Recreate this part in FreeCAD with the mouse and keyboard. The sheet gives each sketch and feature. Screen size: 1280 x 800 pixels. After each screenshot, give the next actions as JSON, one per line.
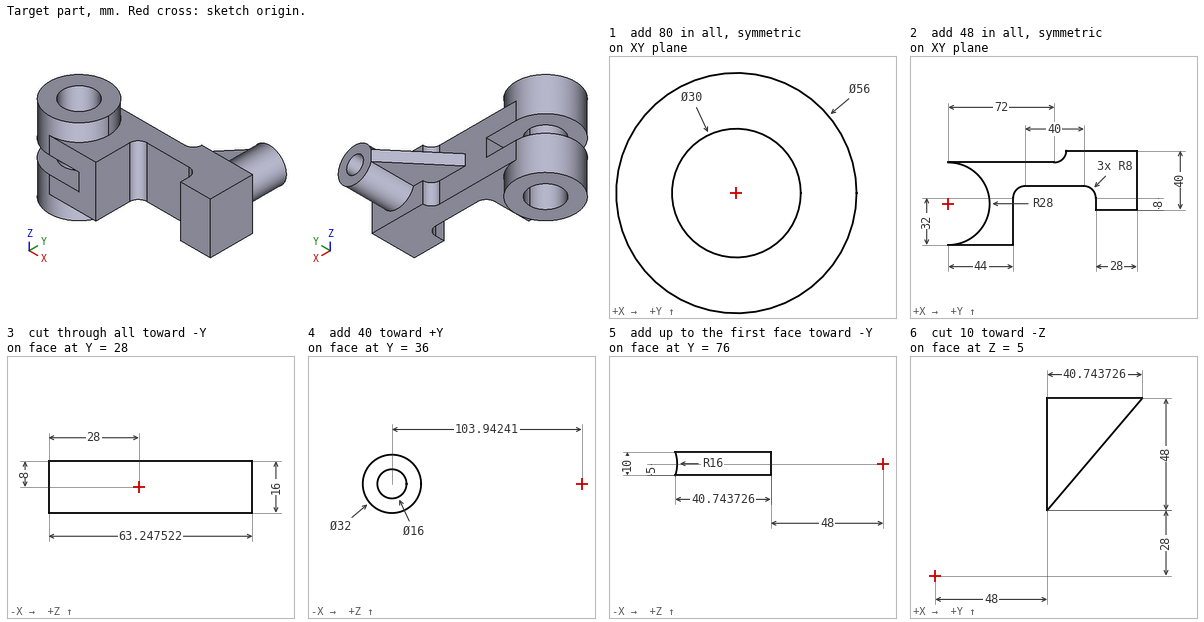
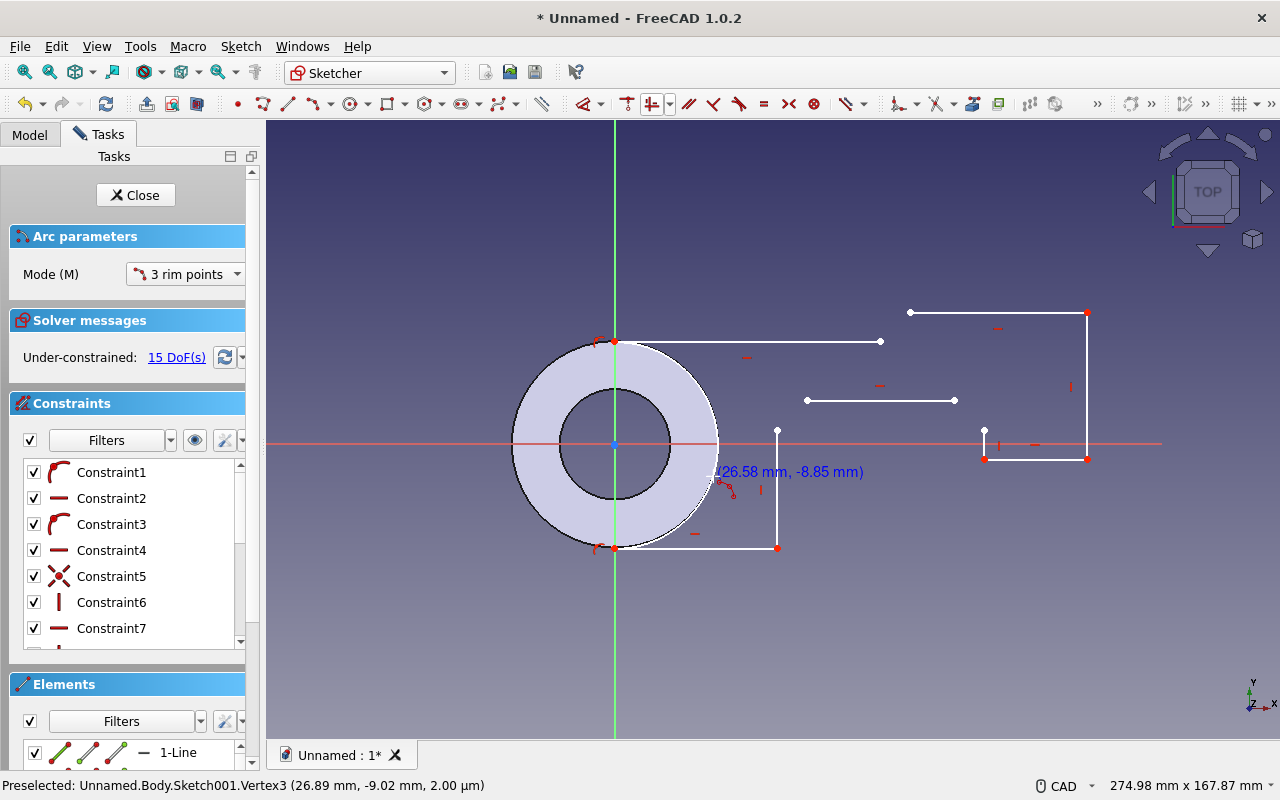
{"action": "left_click", "coordinate": [777, 431]}
{"action": "left_click", "coordinate": [807, 401]}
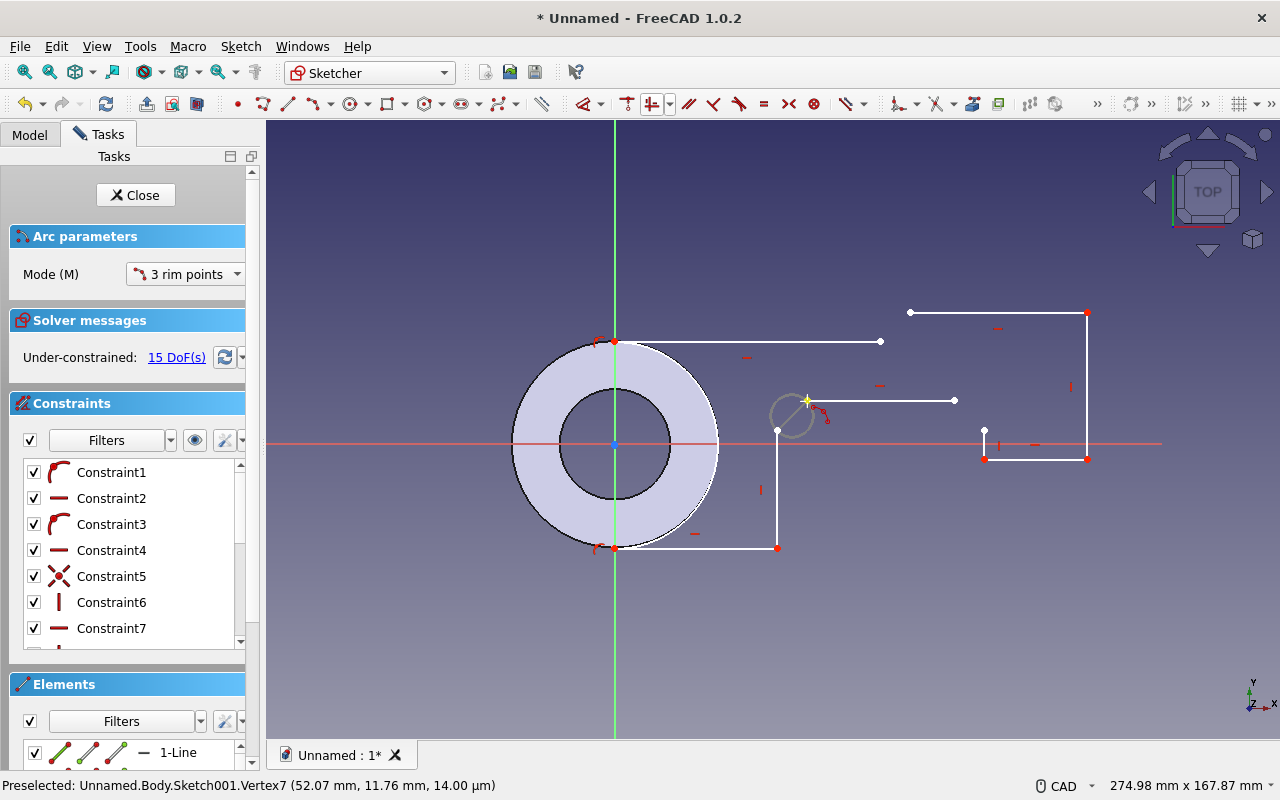
{"action": "scroll", "coordinate": [786, 409], "scroll_direction": "up", "scroll_amount": 4}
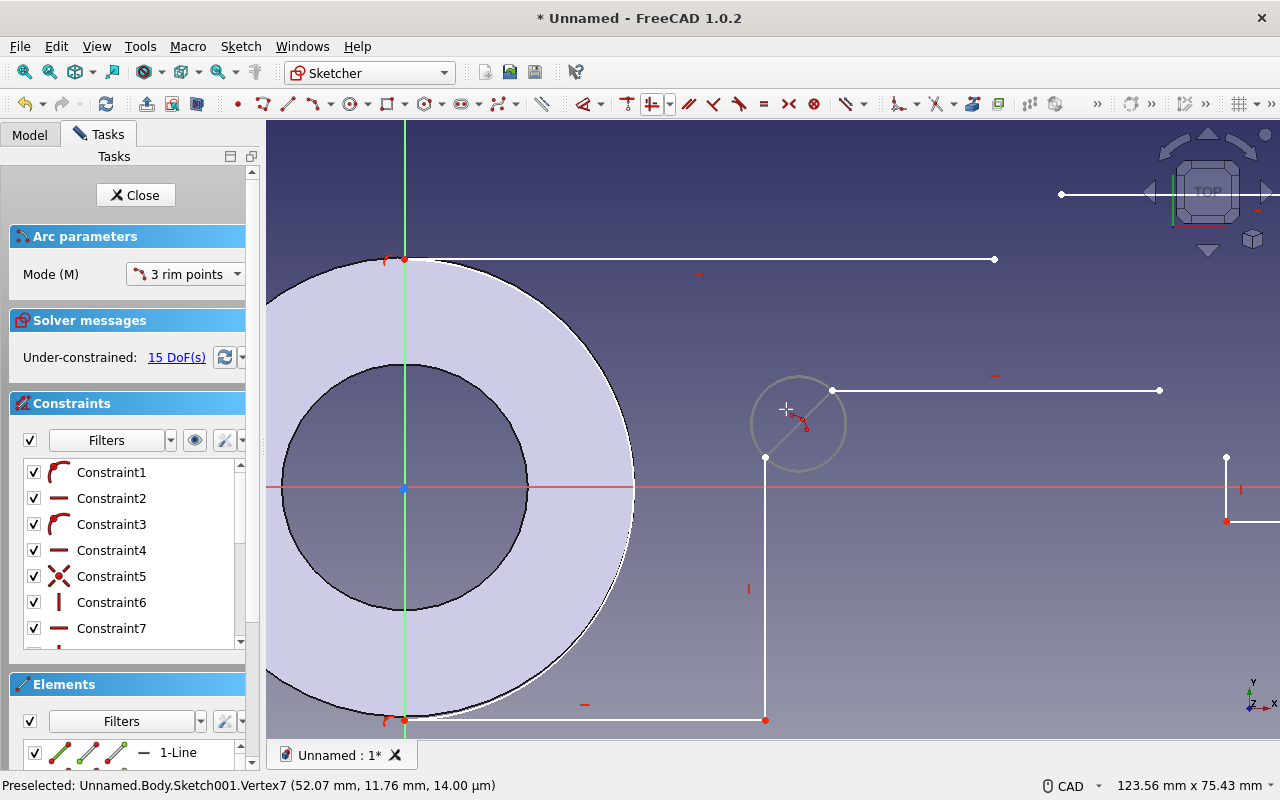
{"action": "left_click", "coordinate": [785, 408]}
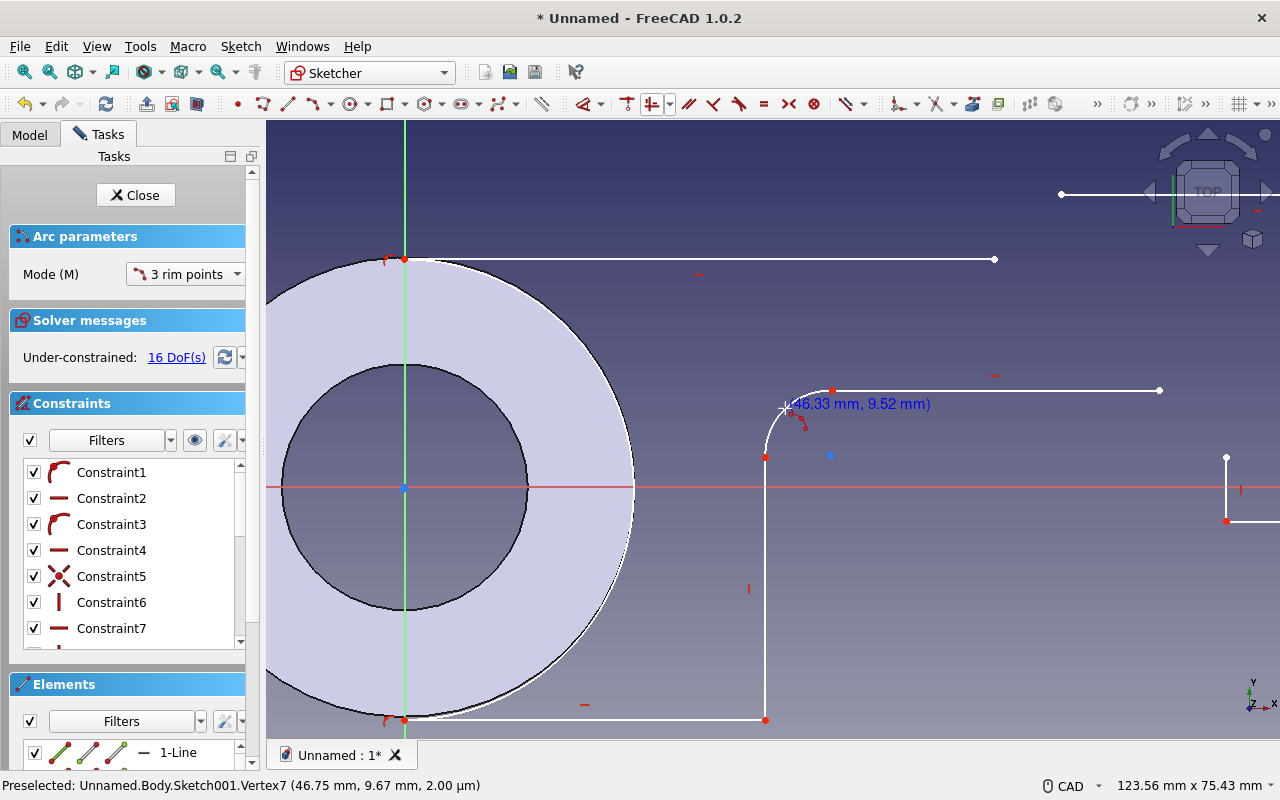
{"action": "scroll", "coordinate": [430, 399], "scroll_direction": "down", "scroll_amount": 3}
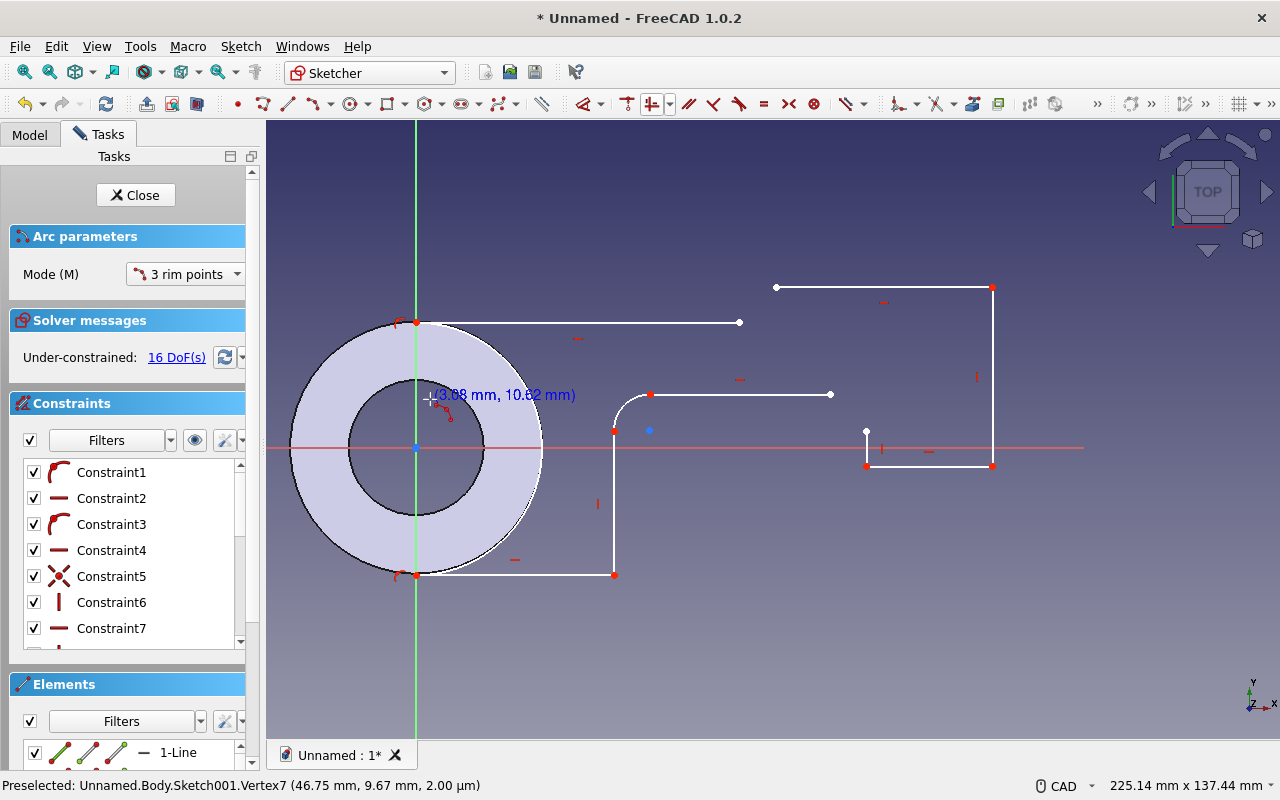
{"action": "left_click", "coordinate": [830, 395]}
{"action": "left_click", "coordinate": [867, 431]}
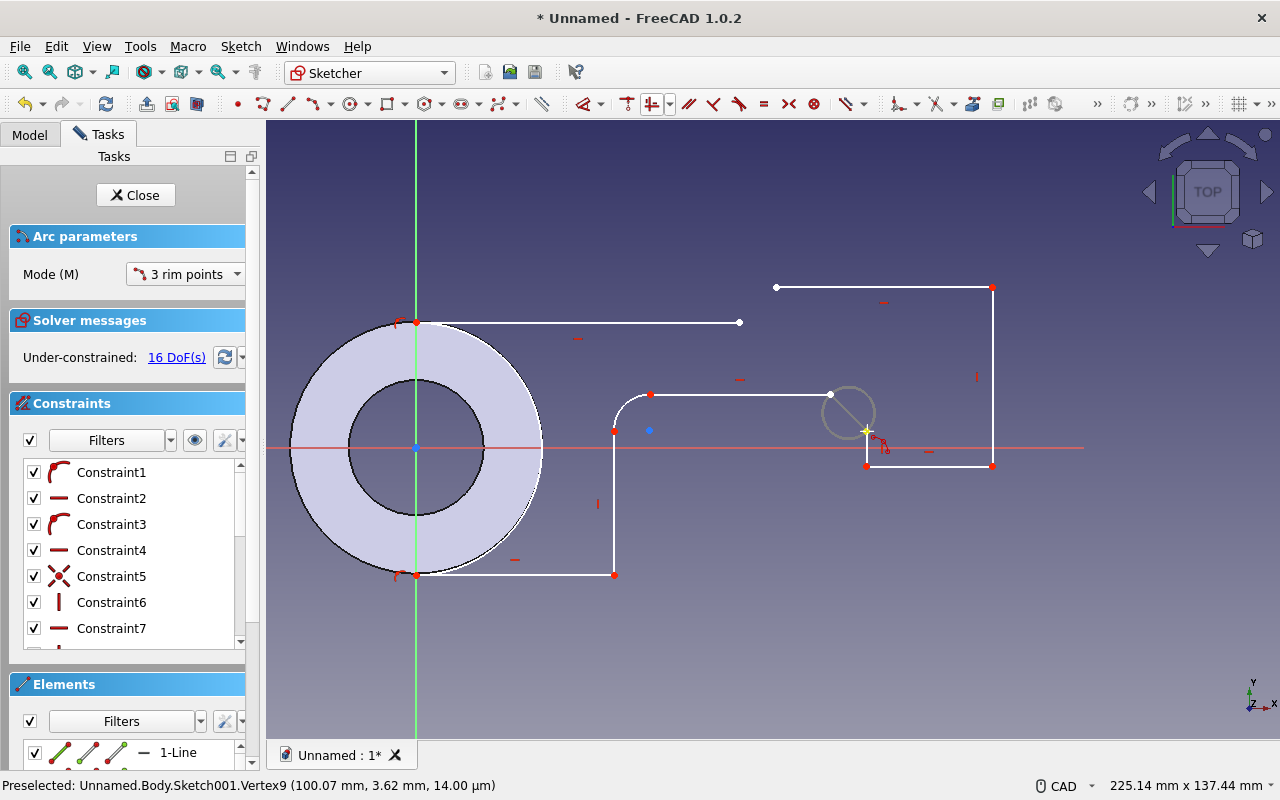
{"action": "scroll", "coordinate": [856, 404], "scroll_direction": "up", "scroll_amount": 3}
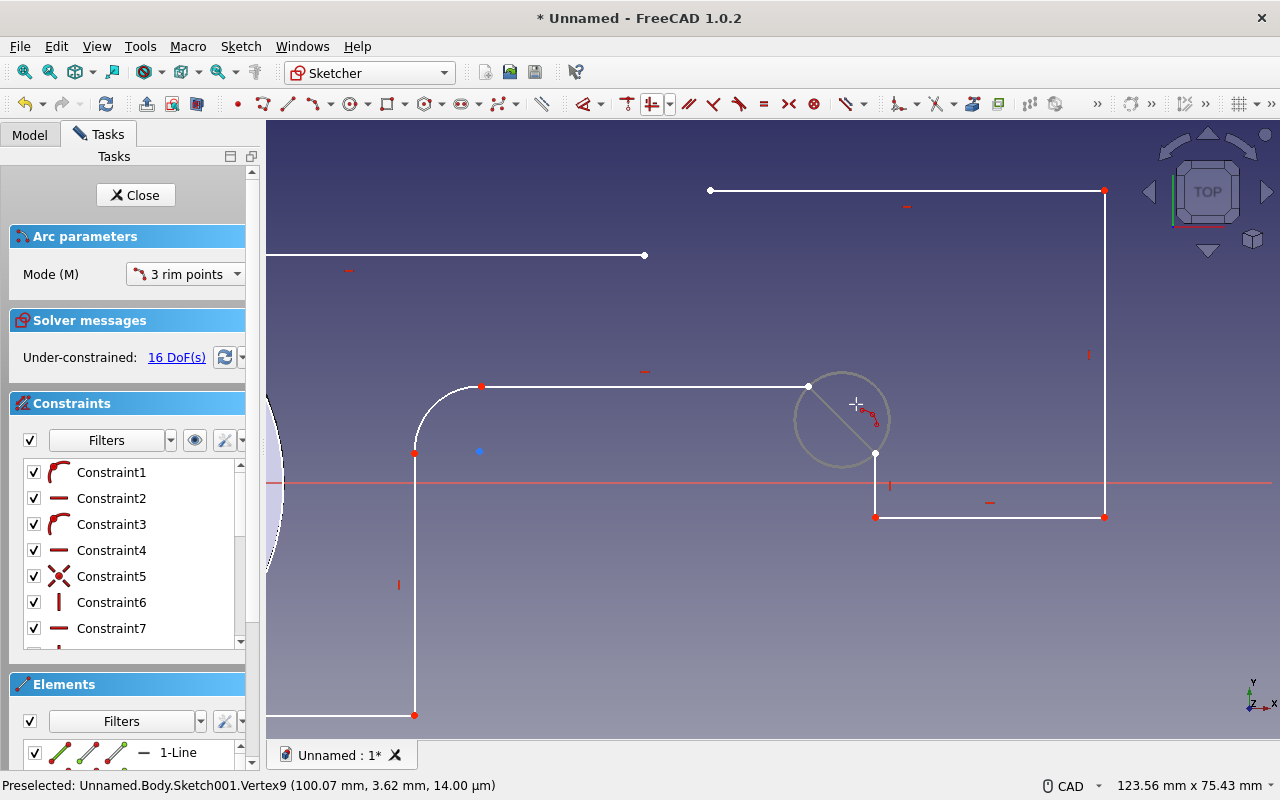
{"action": "left_click", "coordinate": [856, 404]}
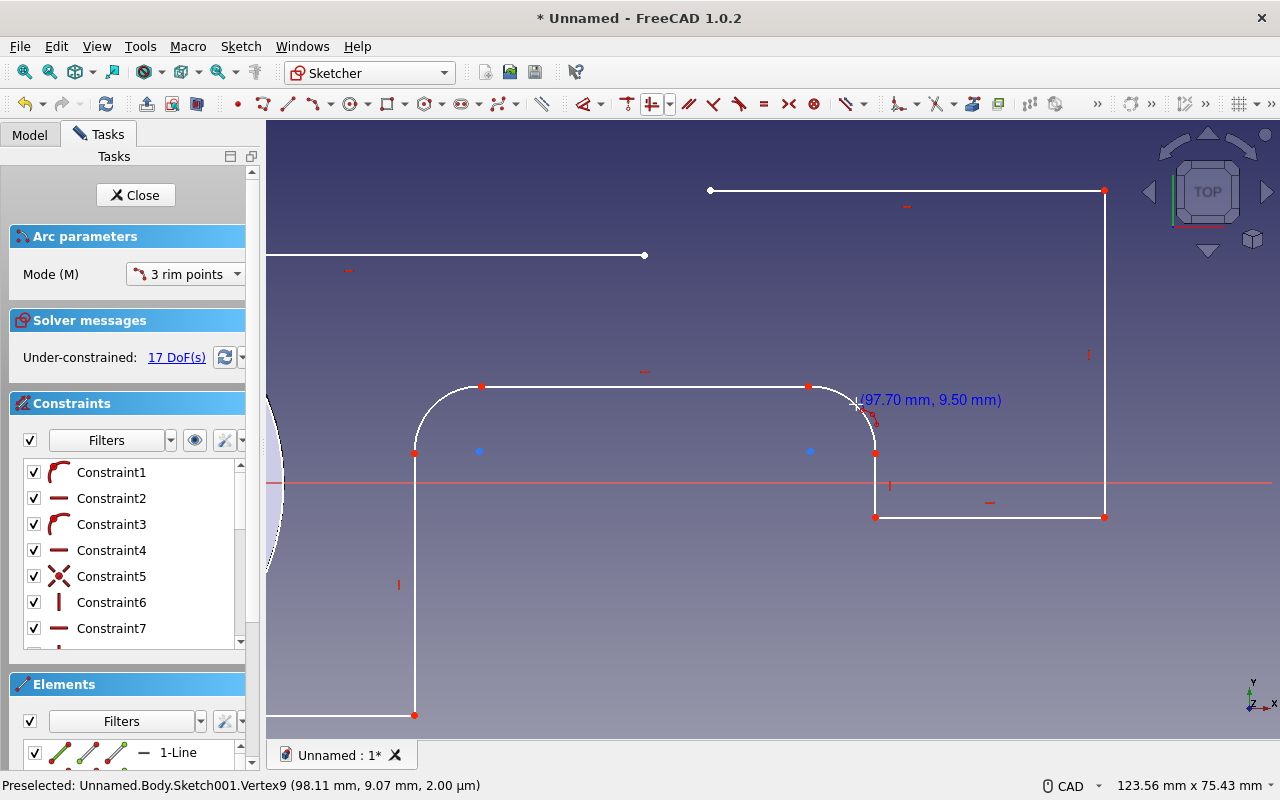
{"action": "left_click", "coordinate": [711, 191]}
{"action": "left_click", "coordinate": [644, 255]}
{"action": "left_click", "coordinate": [691, 234]}
{"action": "key", "text": "Escape"}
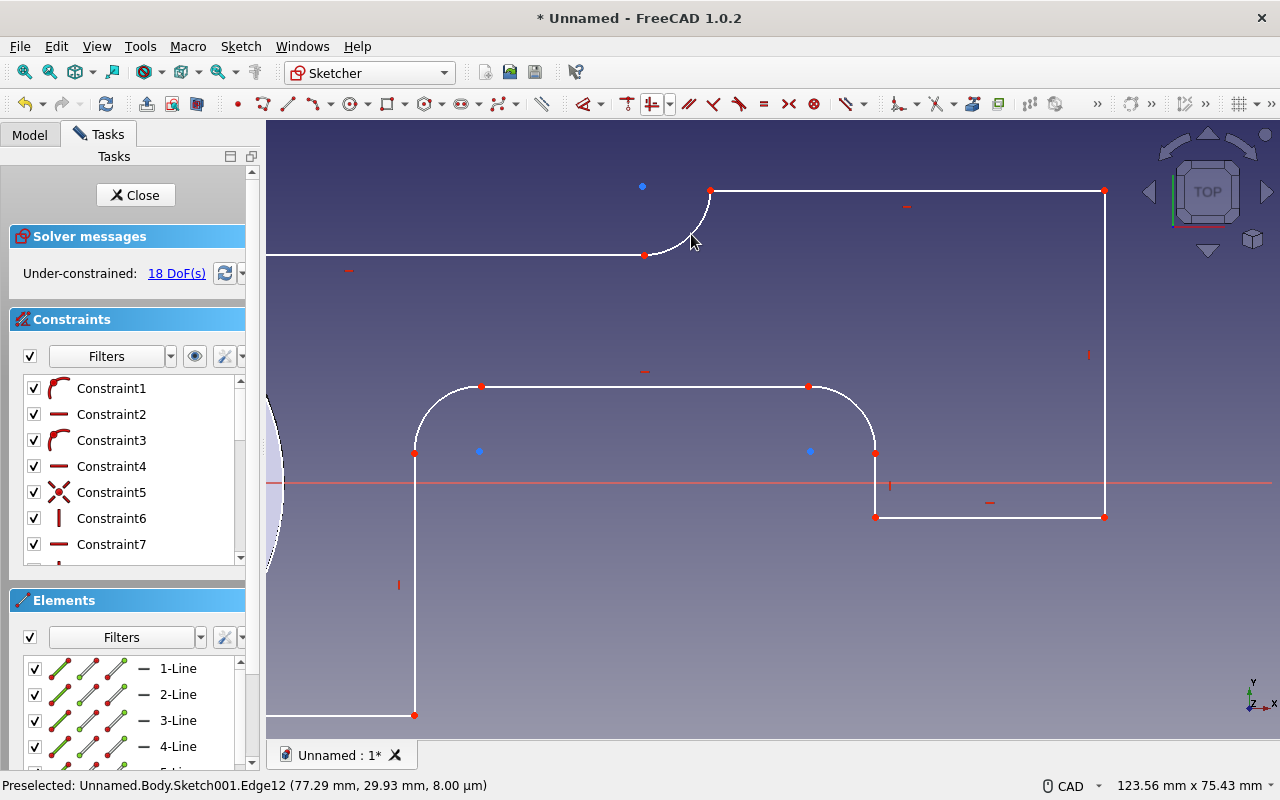
{"action": "left_click", "coordinate": [467, 255]}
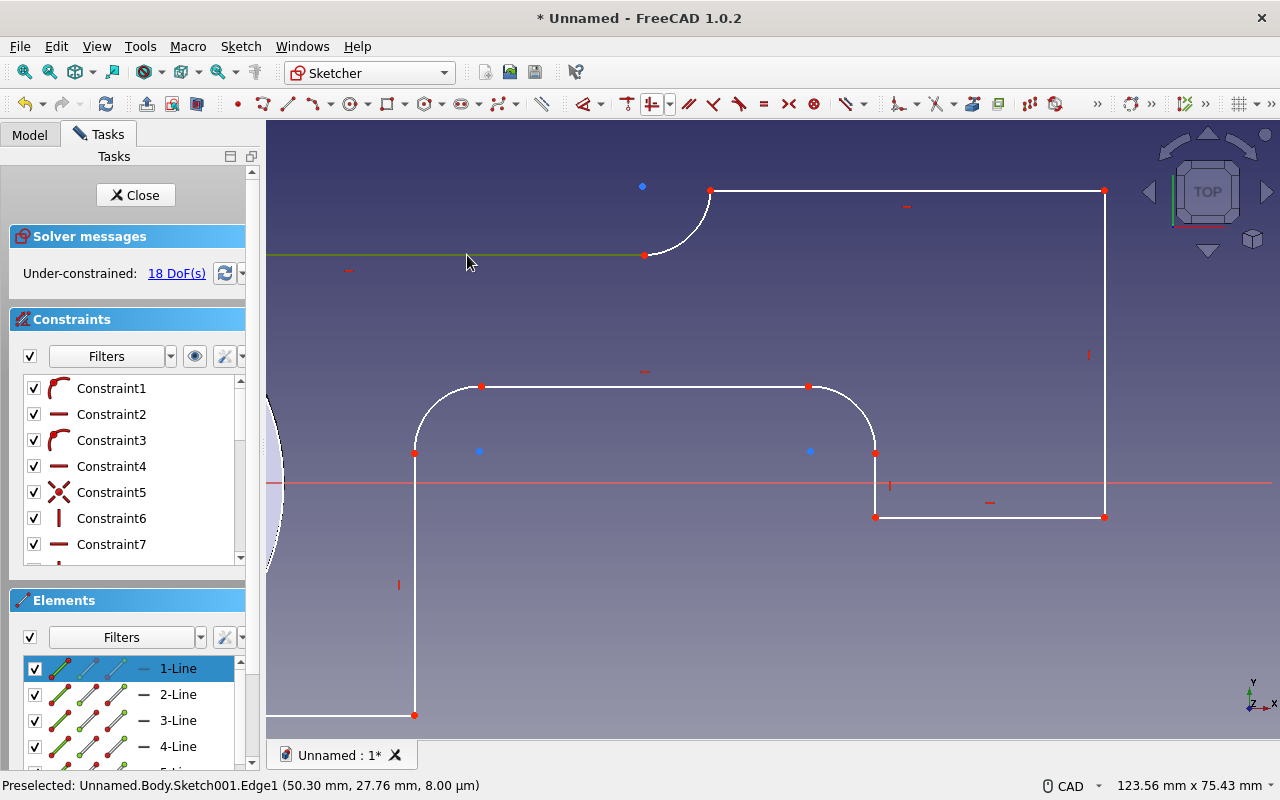
{"action": "scroll", "coordinate": [857, 404], "scroll_direction": "down", "scroll_amount": 3}